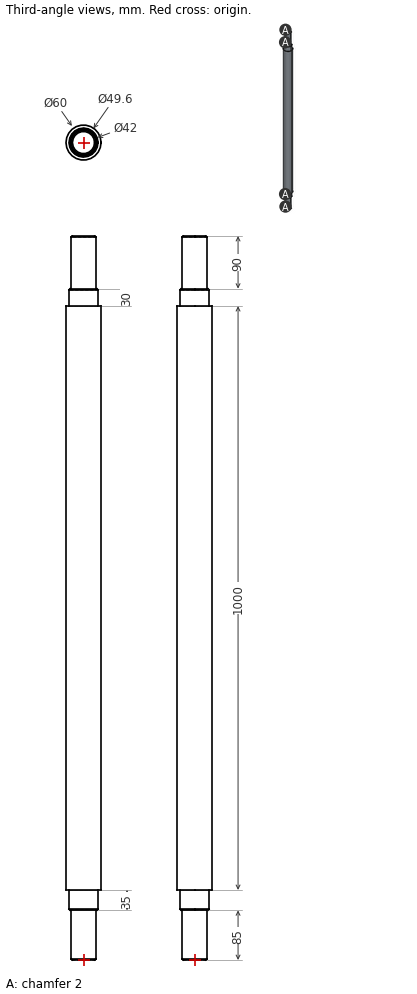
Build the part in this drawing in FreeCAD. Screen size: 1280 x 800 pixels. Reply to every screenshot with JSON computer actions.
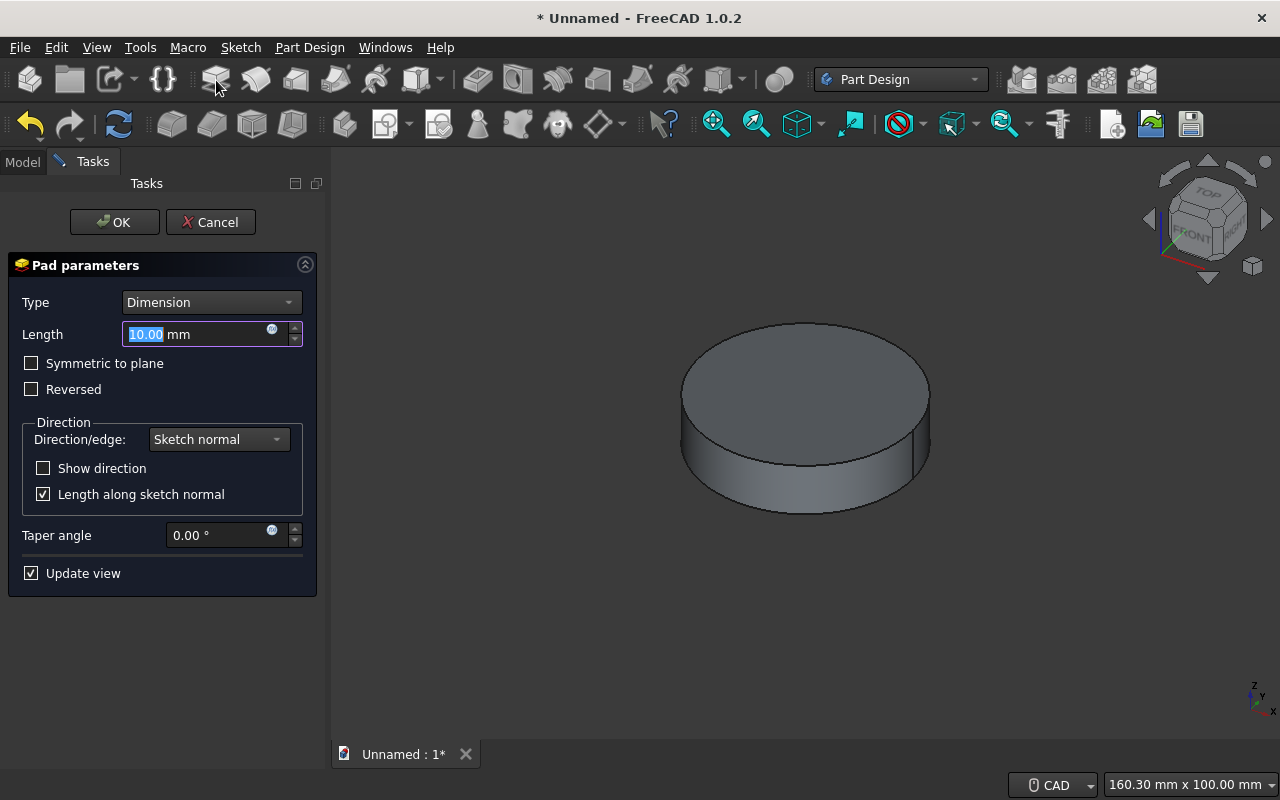
{"action": "type", "text": "85"}
{"action": "key", "text": "Tab"}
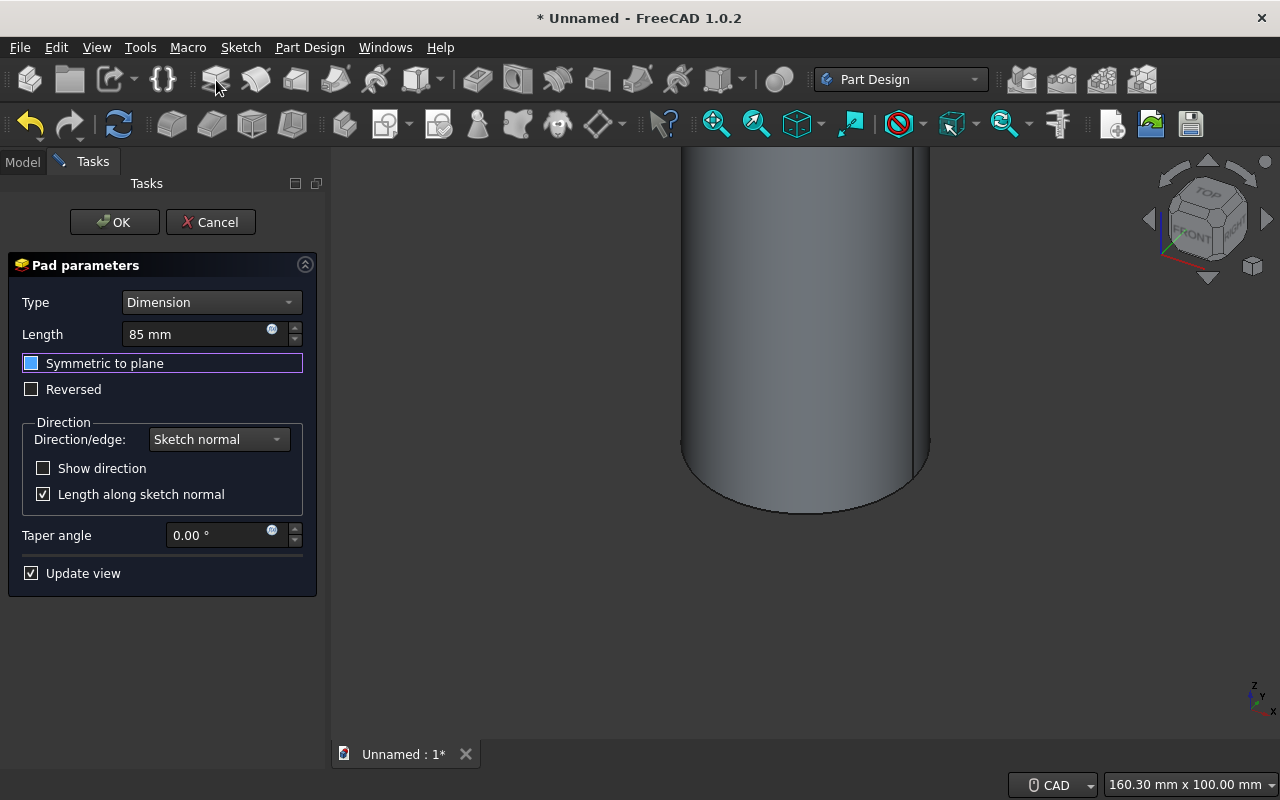
{"action": "left_click", "coordinate": [115, 222]}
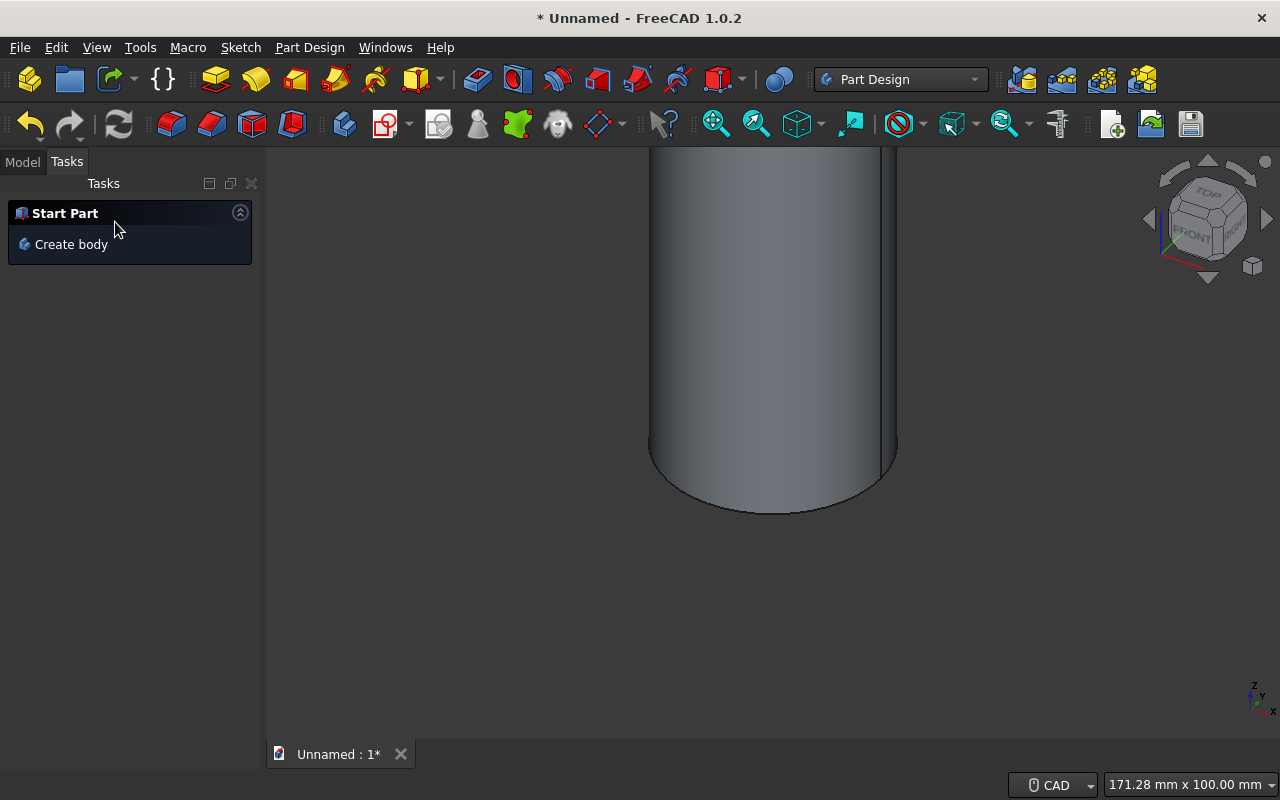
{"action": "left_click", "coordinate": [718, 124]}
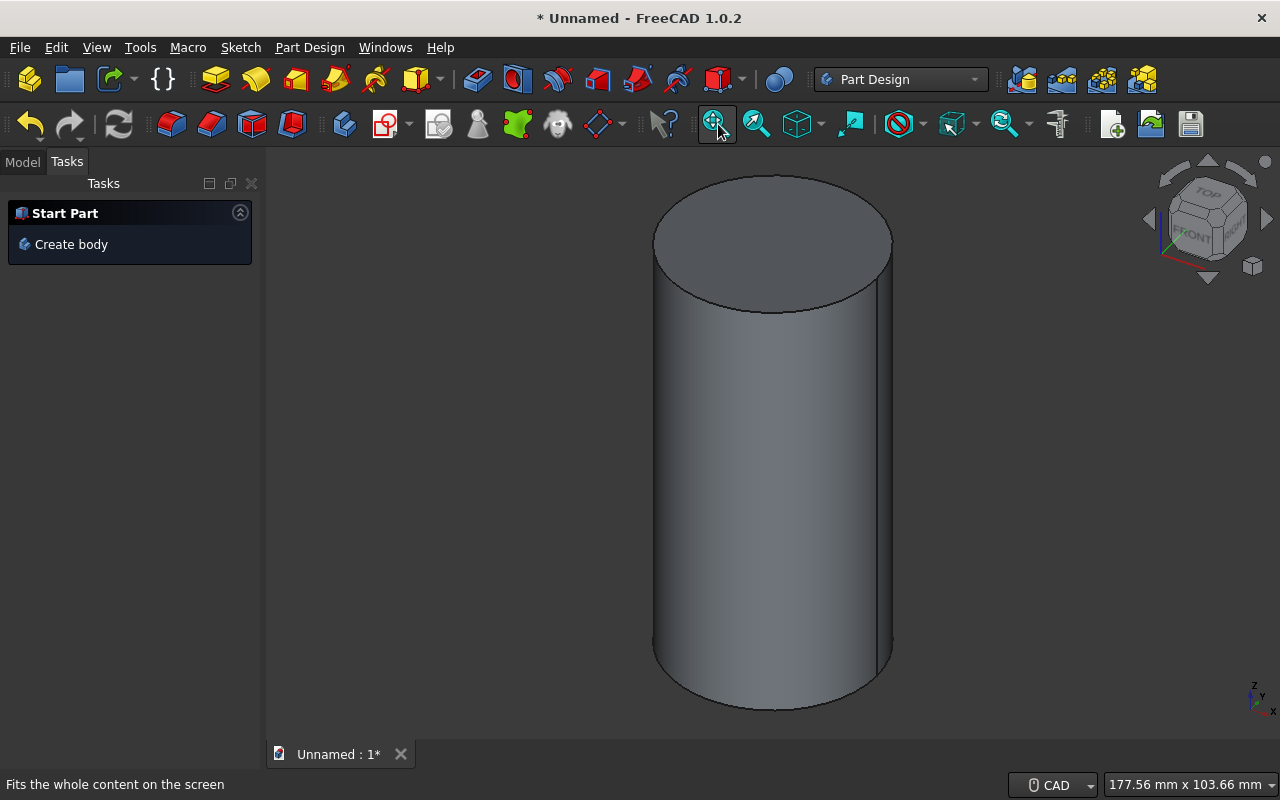
{"action": "left_click", "coordinate": [773, 243]}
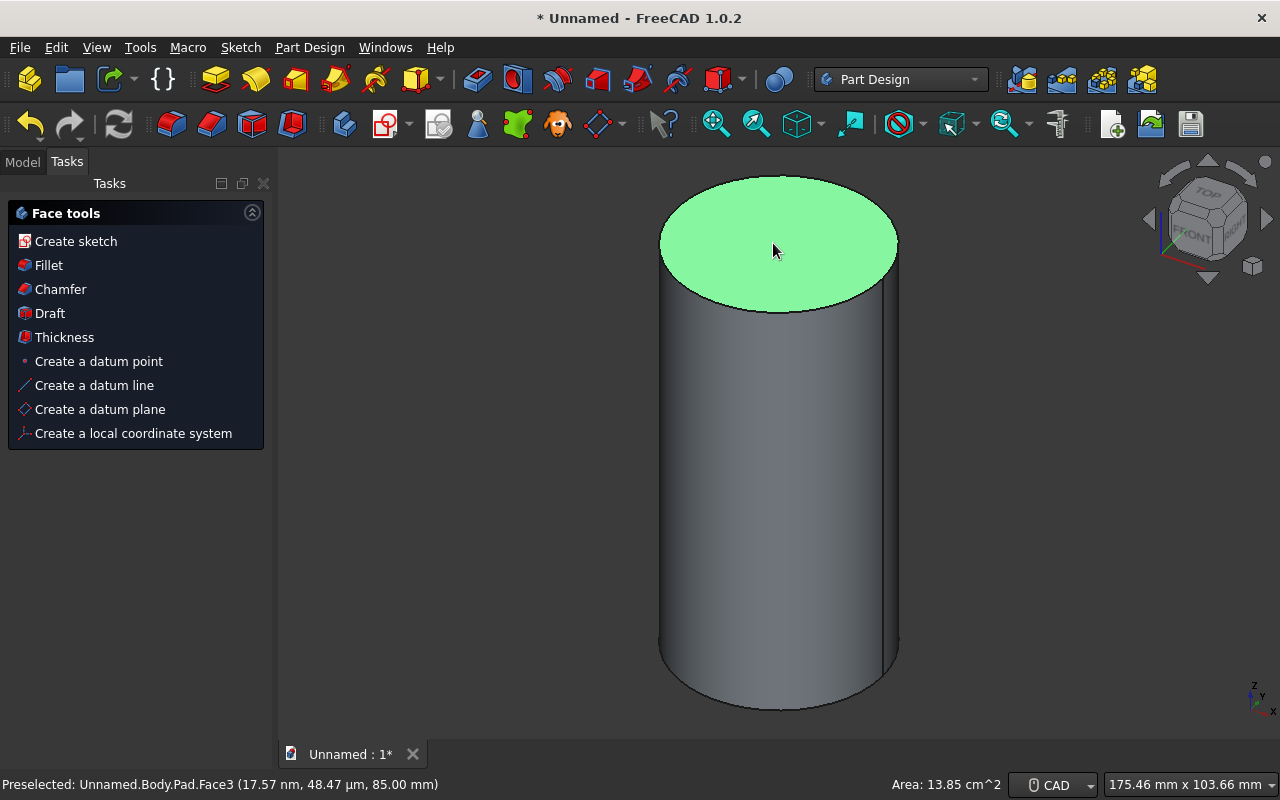
{"action": "left_click", "coordinate": [386, 124]}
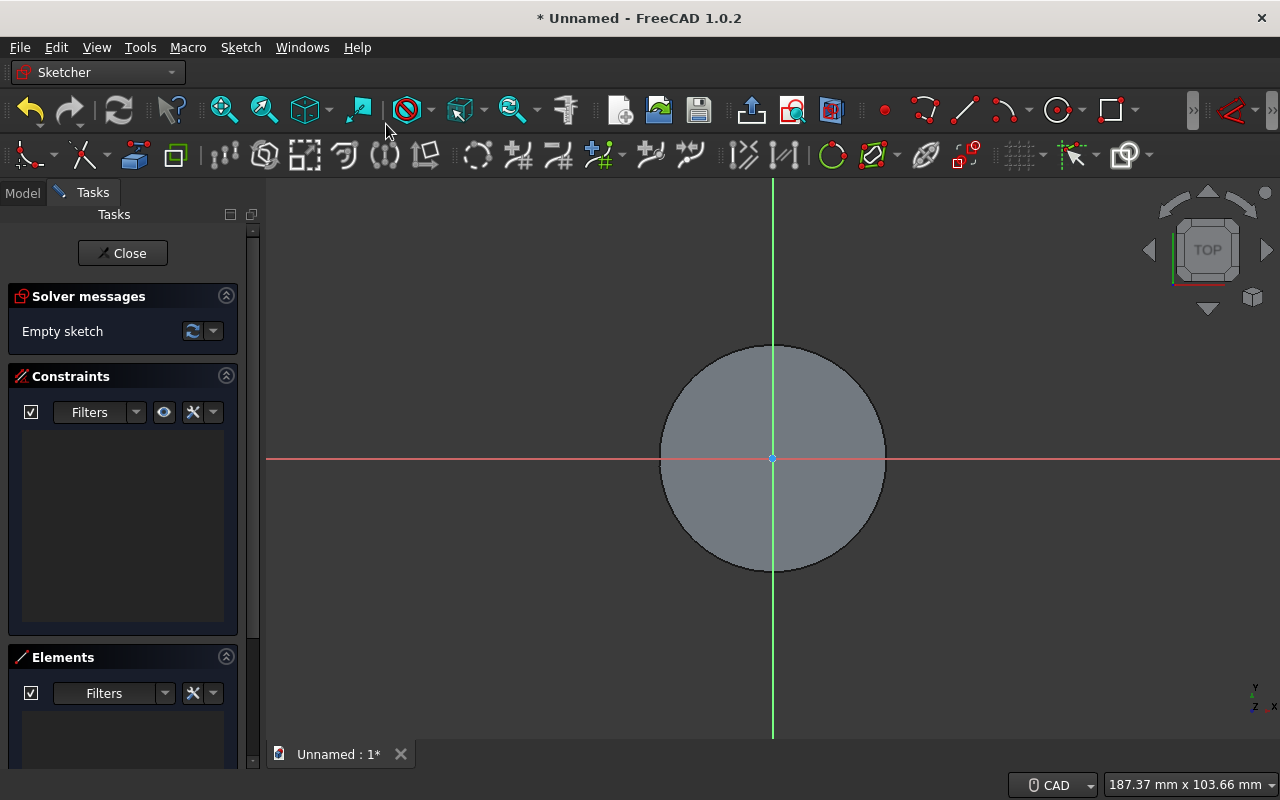
{"action": "key", "text": "g c"}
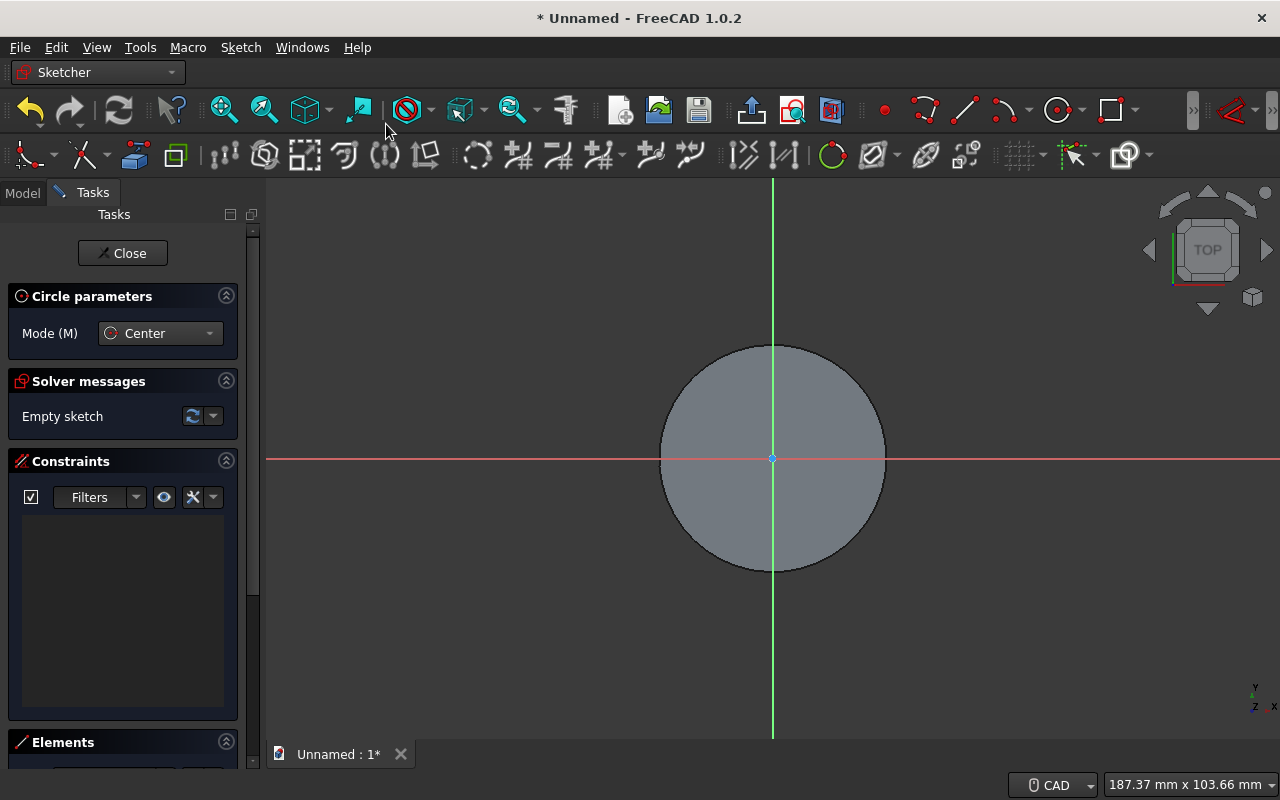
{"action": "left_click", "coordinate": [773, 458]}
{"action": "mouse_move", "coordinate": [868, 364]}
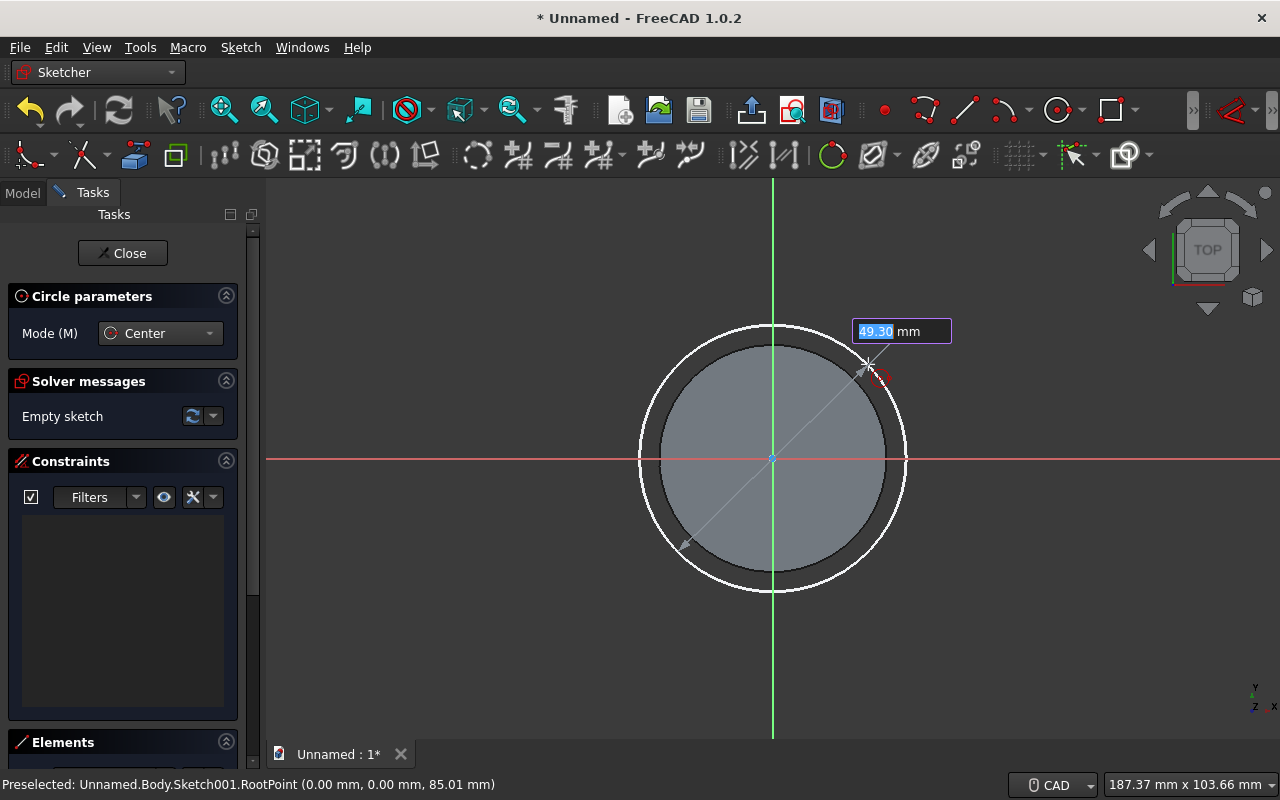
{"action": "type", "text": "49.6"}
{"action": "key", "text": "Return"}
{"action": "key", "text": "Escape"}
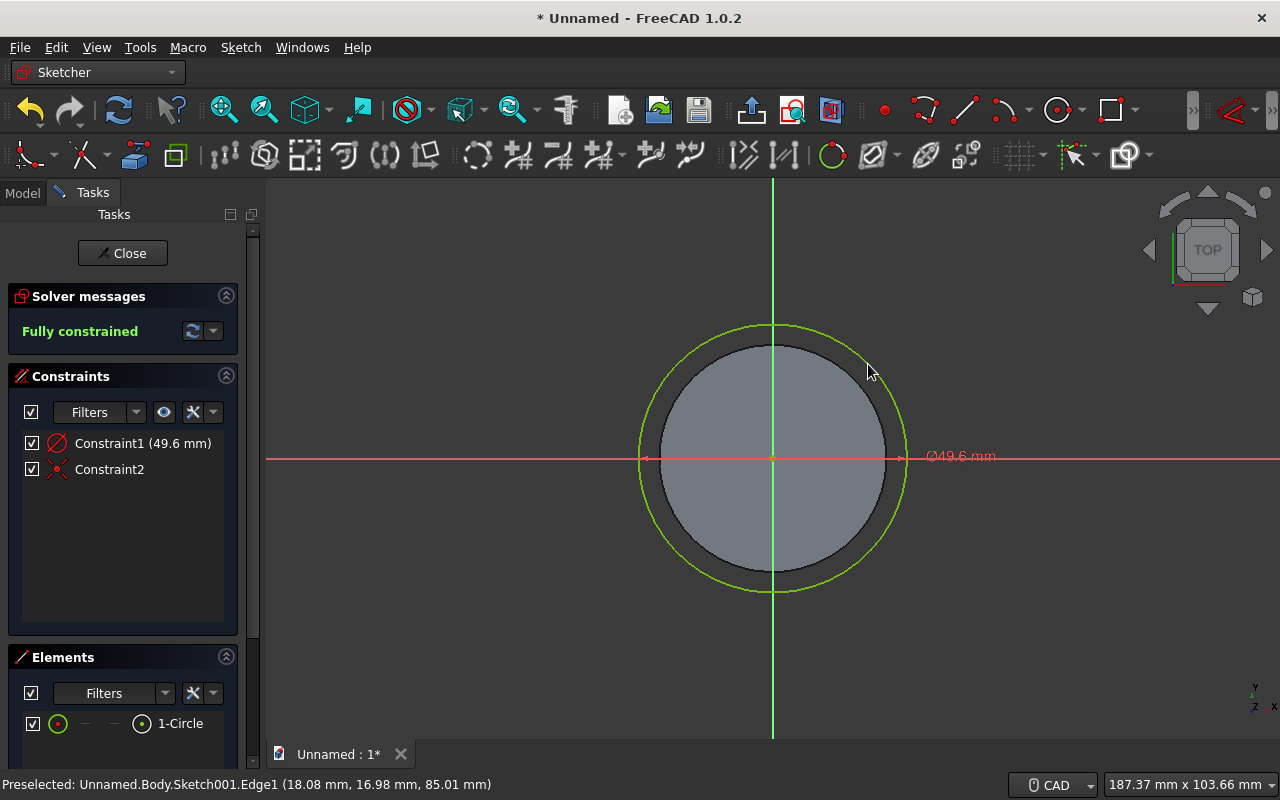
{"action": "left_click", "coordinate": [123, 253]}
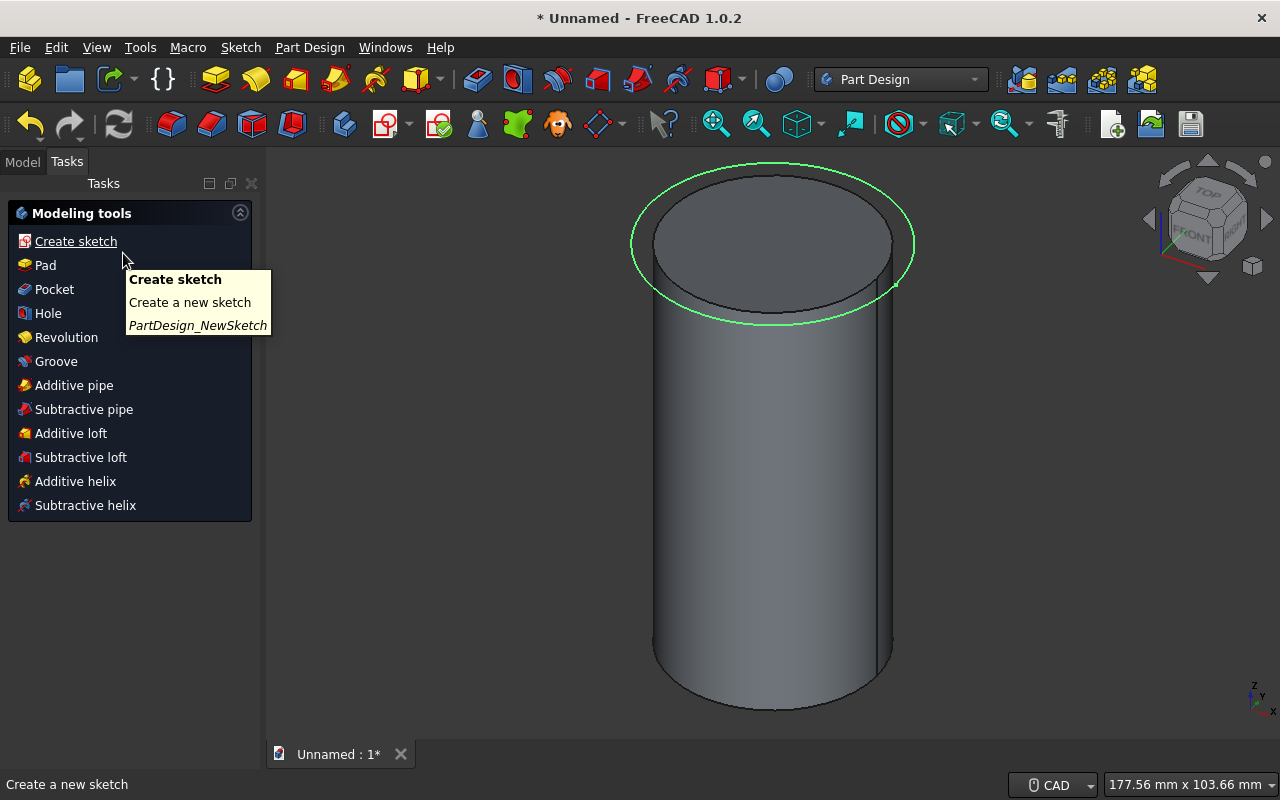
{"action": "left_click", "coordinate": [216, 80]}